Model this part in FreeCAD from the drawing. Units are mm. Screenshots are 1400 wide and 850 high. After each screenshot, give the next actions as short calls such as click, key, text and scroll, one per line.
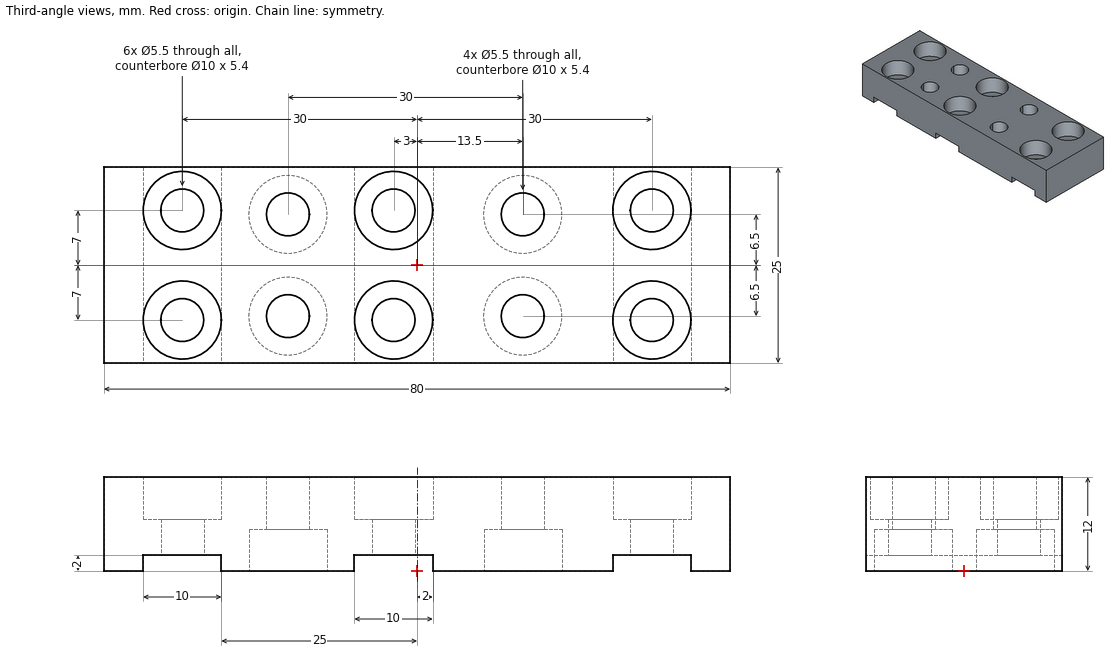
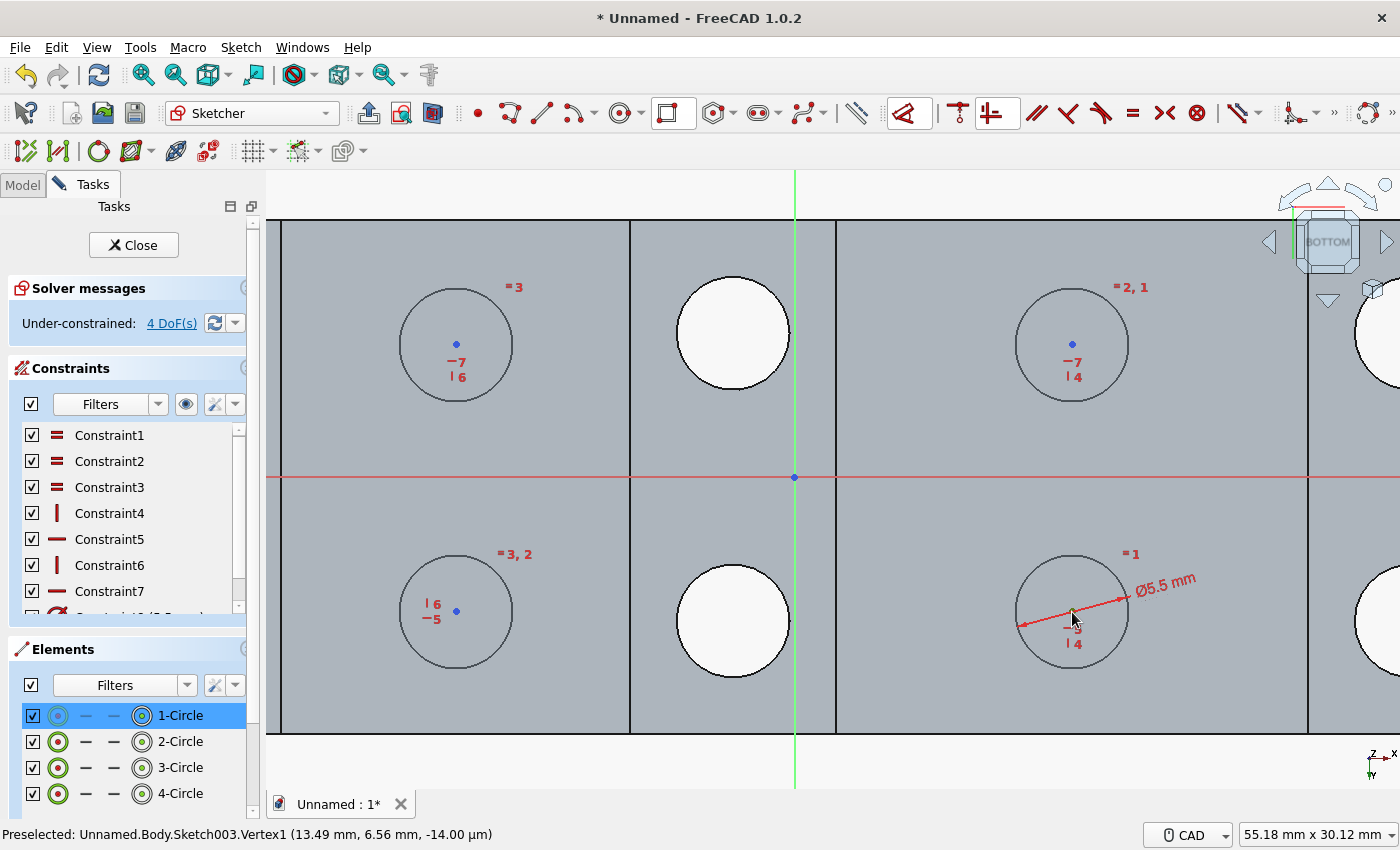
key(i)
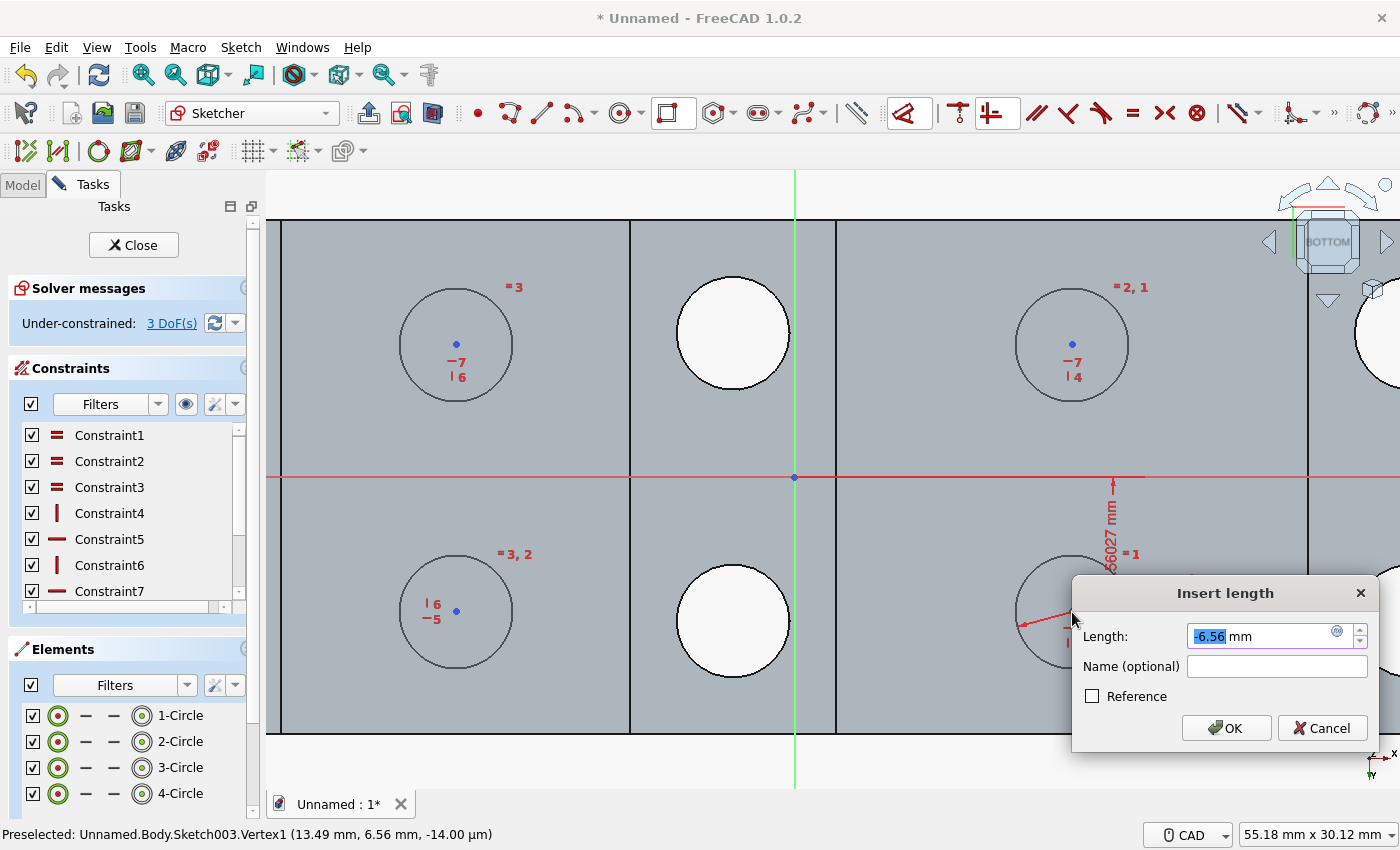
text(-6.5)
key(Return)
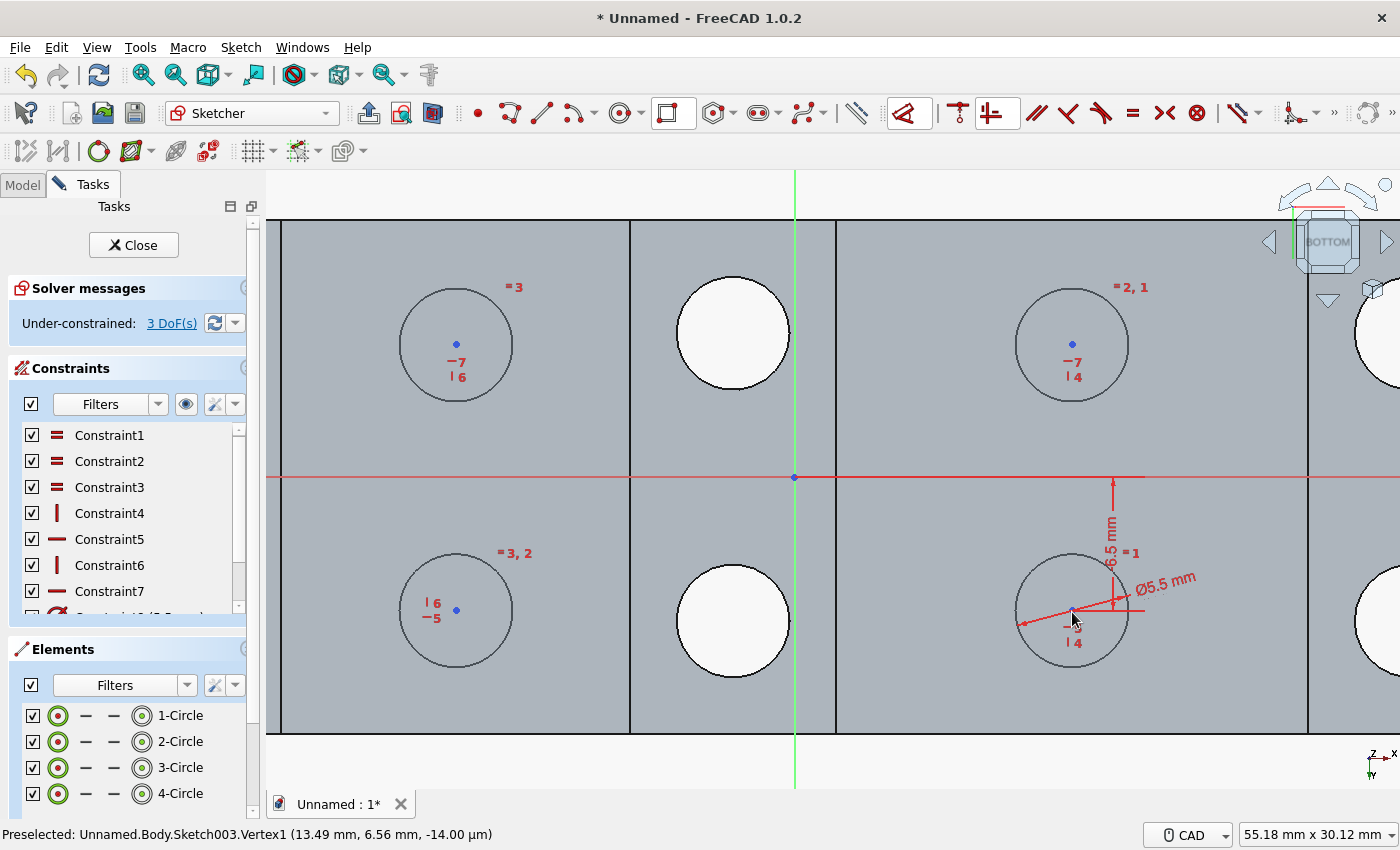
click(1072, 345)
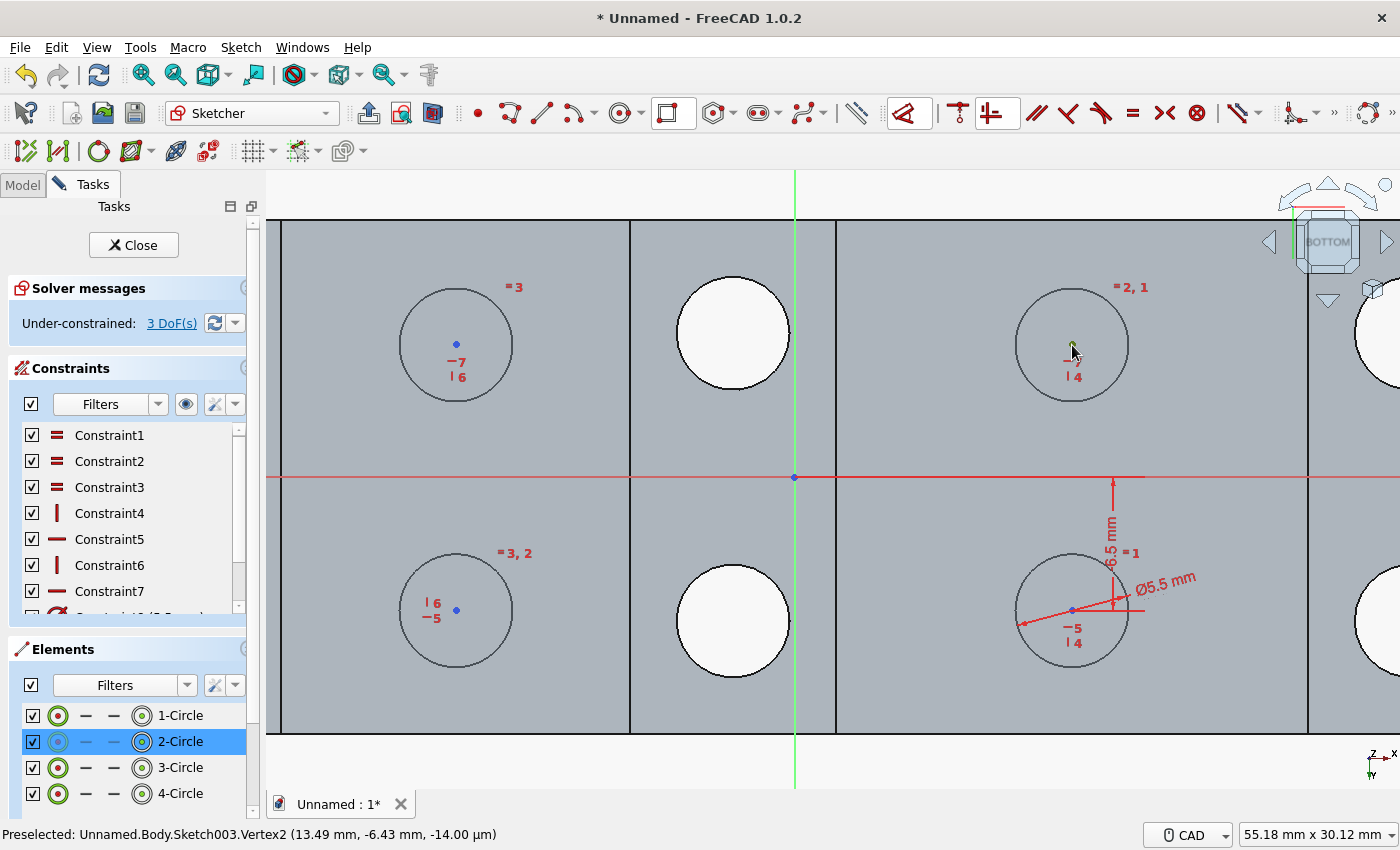
key(i)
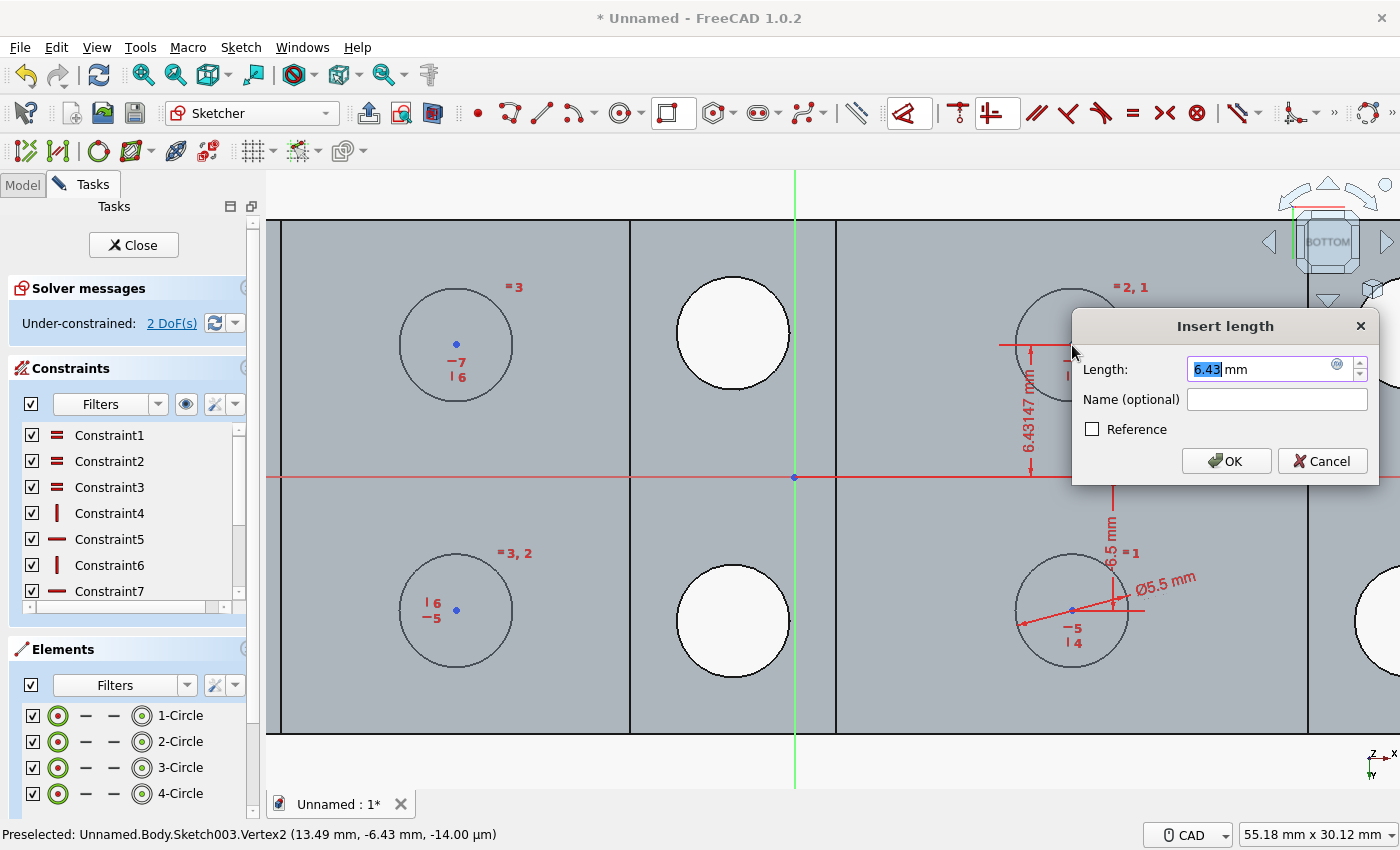
text(6.5)
key(Return)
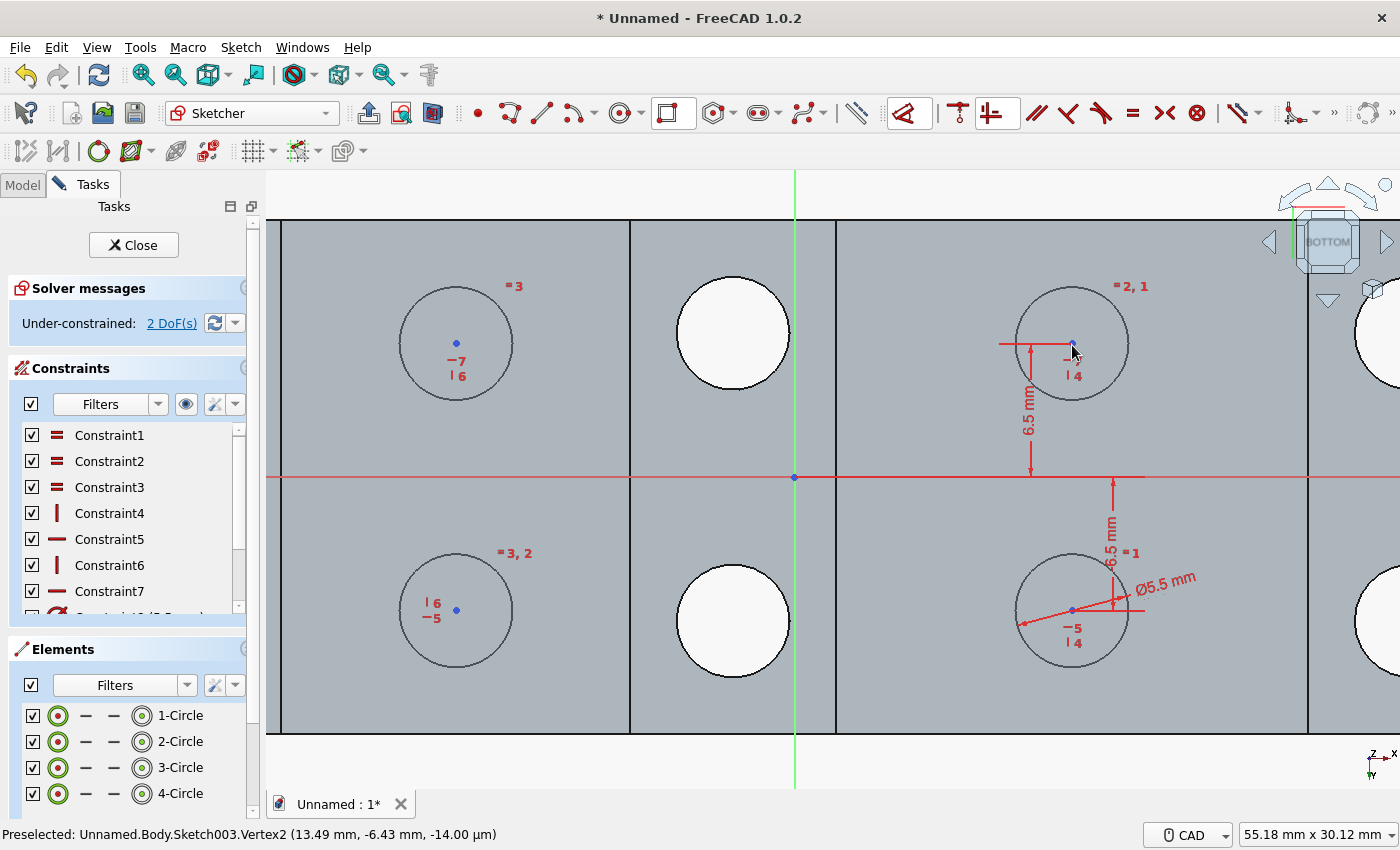
click(1072, 611)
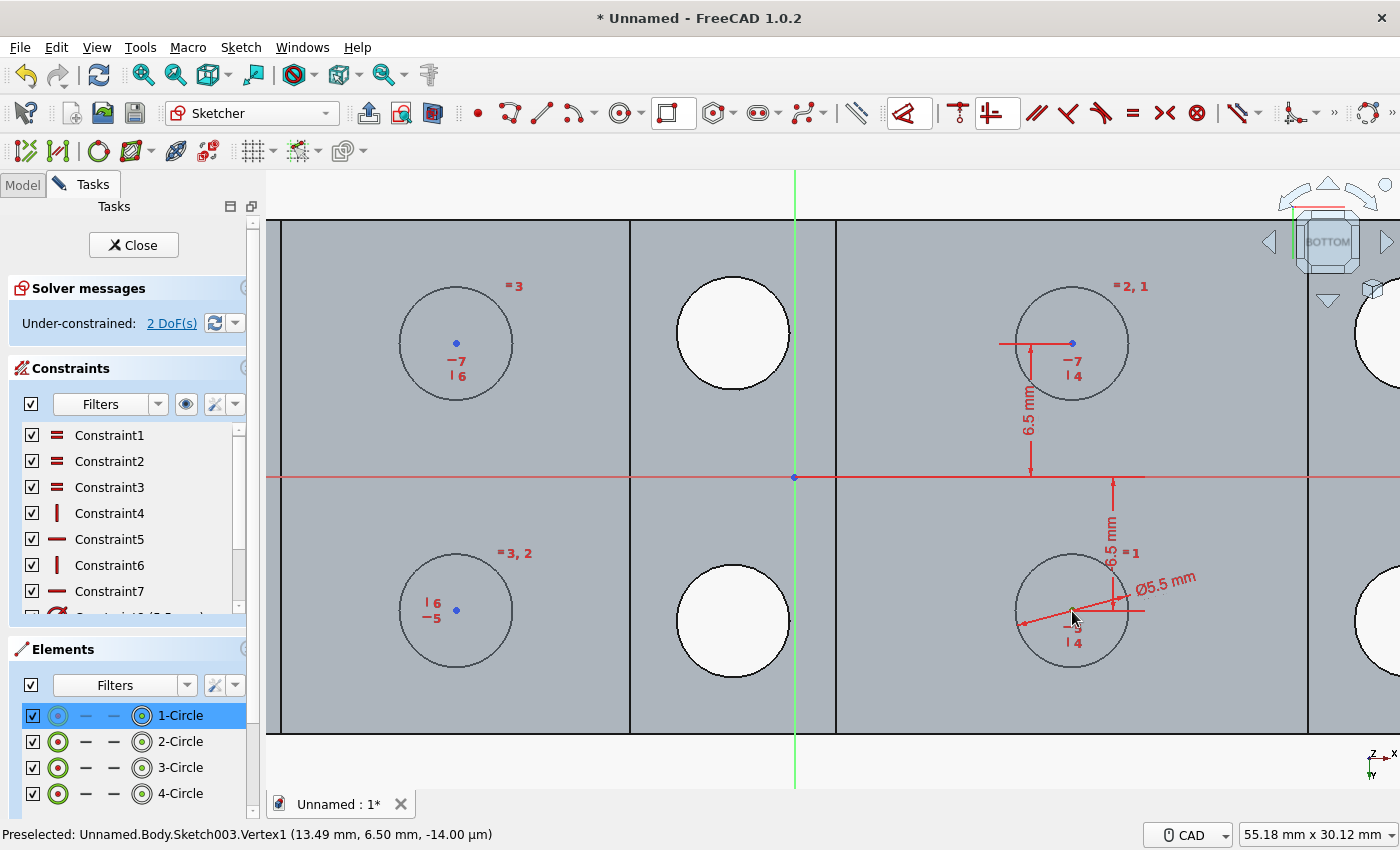
click(456, 611)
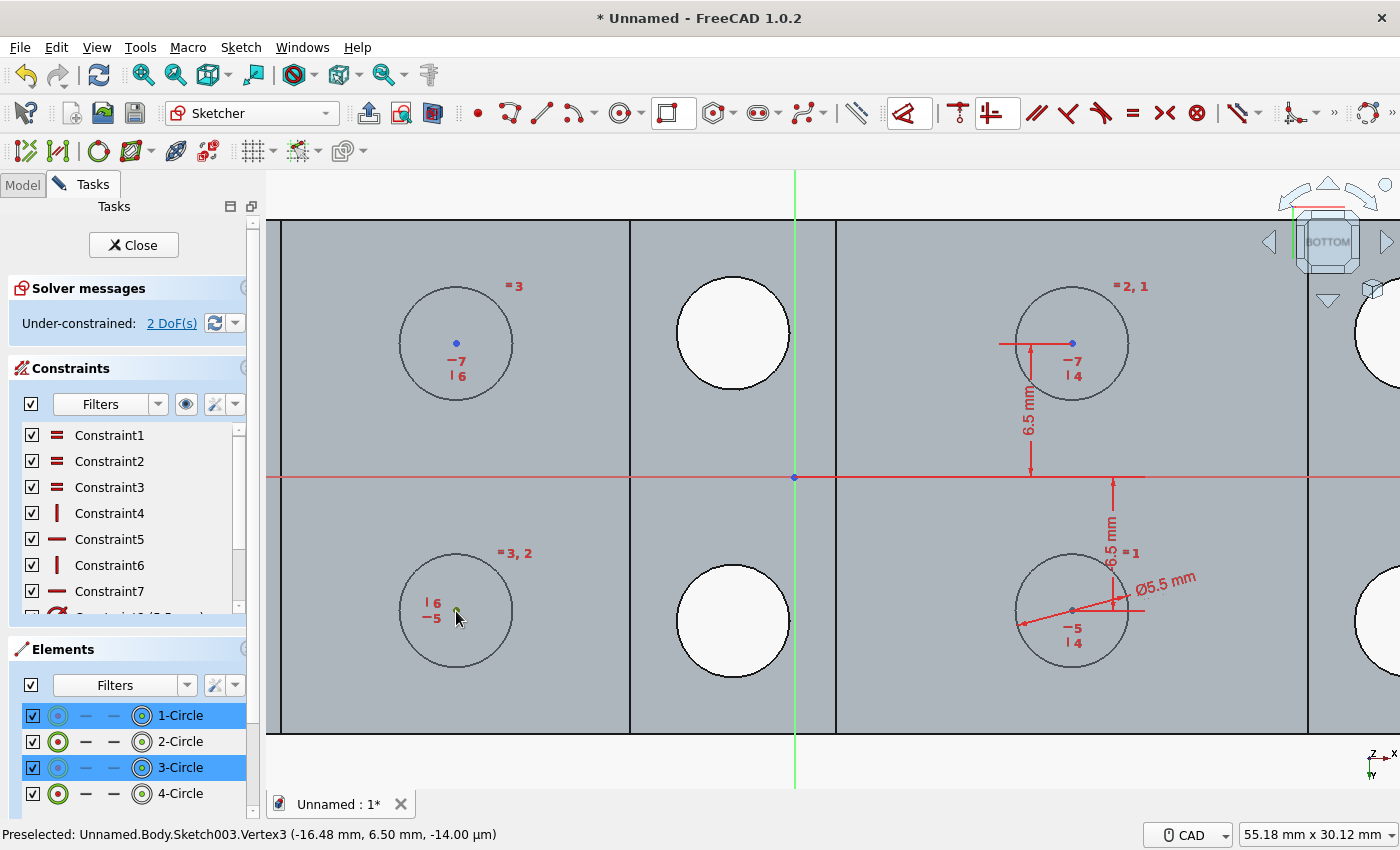
key(l)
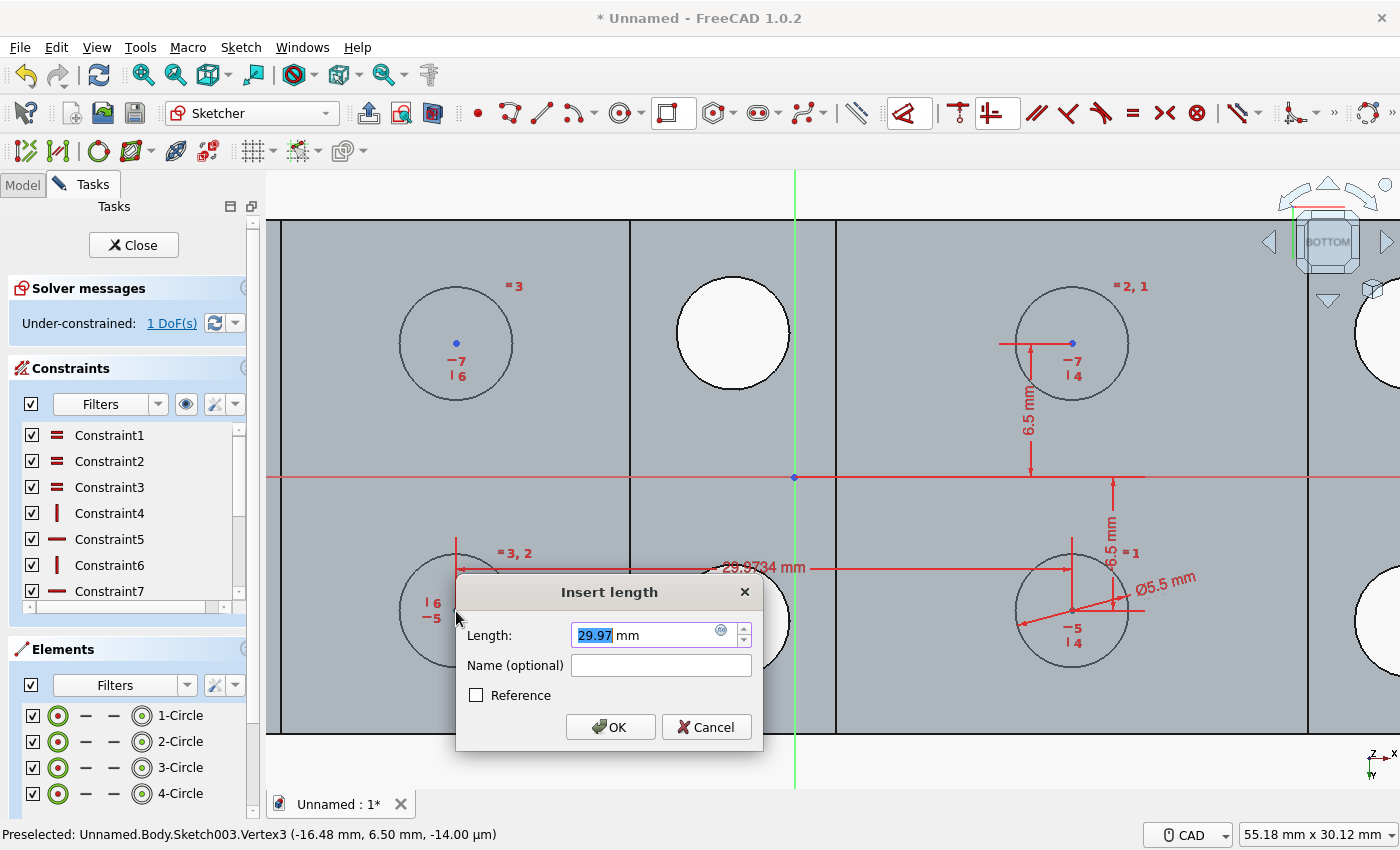
text(30)
key(Return)